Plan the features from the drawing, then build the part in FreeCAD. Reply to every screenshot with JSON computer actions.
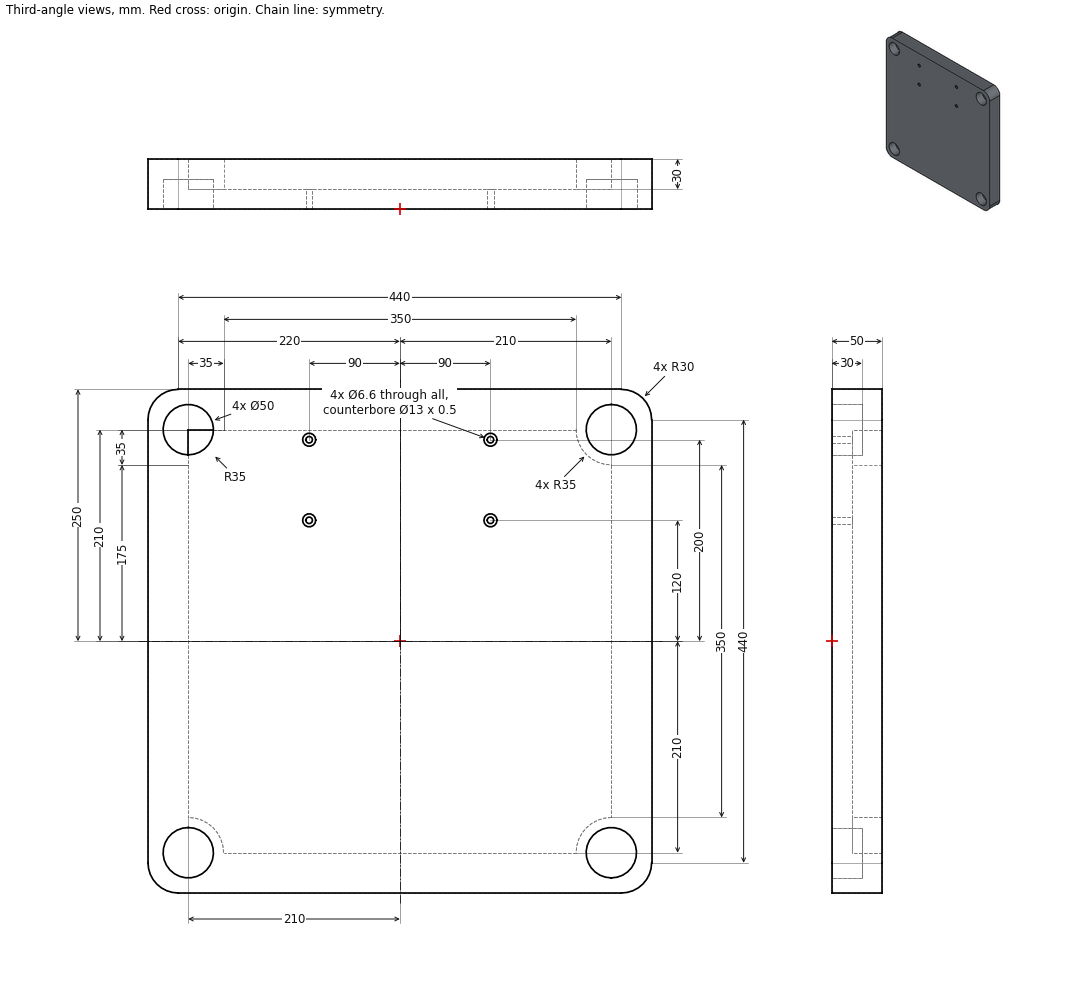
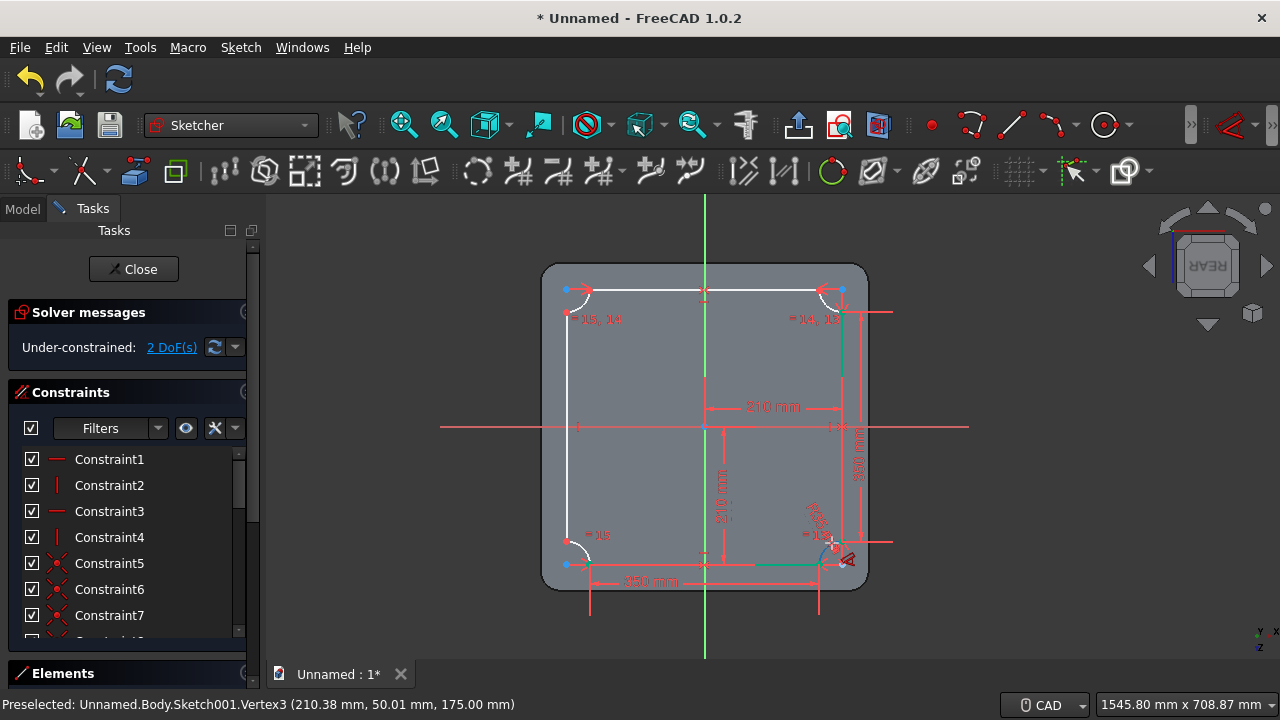
{"action": "left_click", "coordinate": [819, 290]}
{"action": "left_click", "coordinate": [671, 359]}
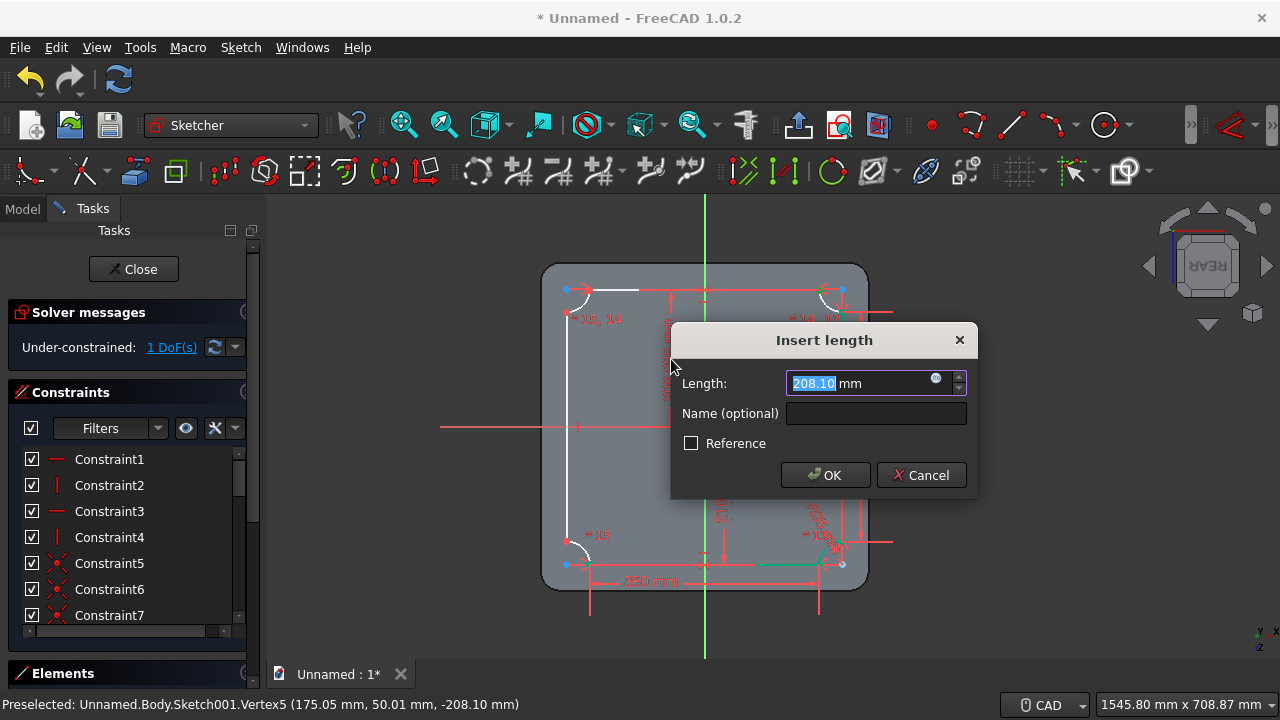
{"action": "type", "text": "210"}
{"action": "key", "text": "Return"}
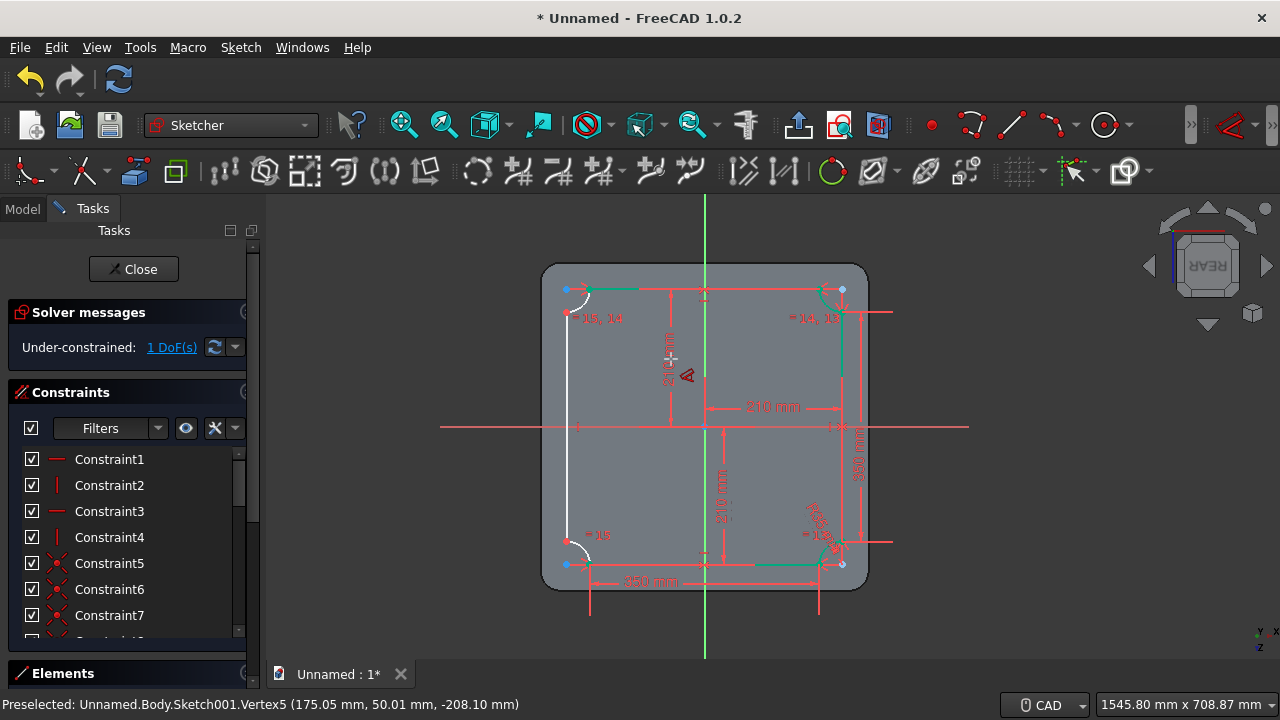
{"action": "left_click", "coordinate": [567, 312]}
{"action": "left_click", "coordinate": [636, 461]}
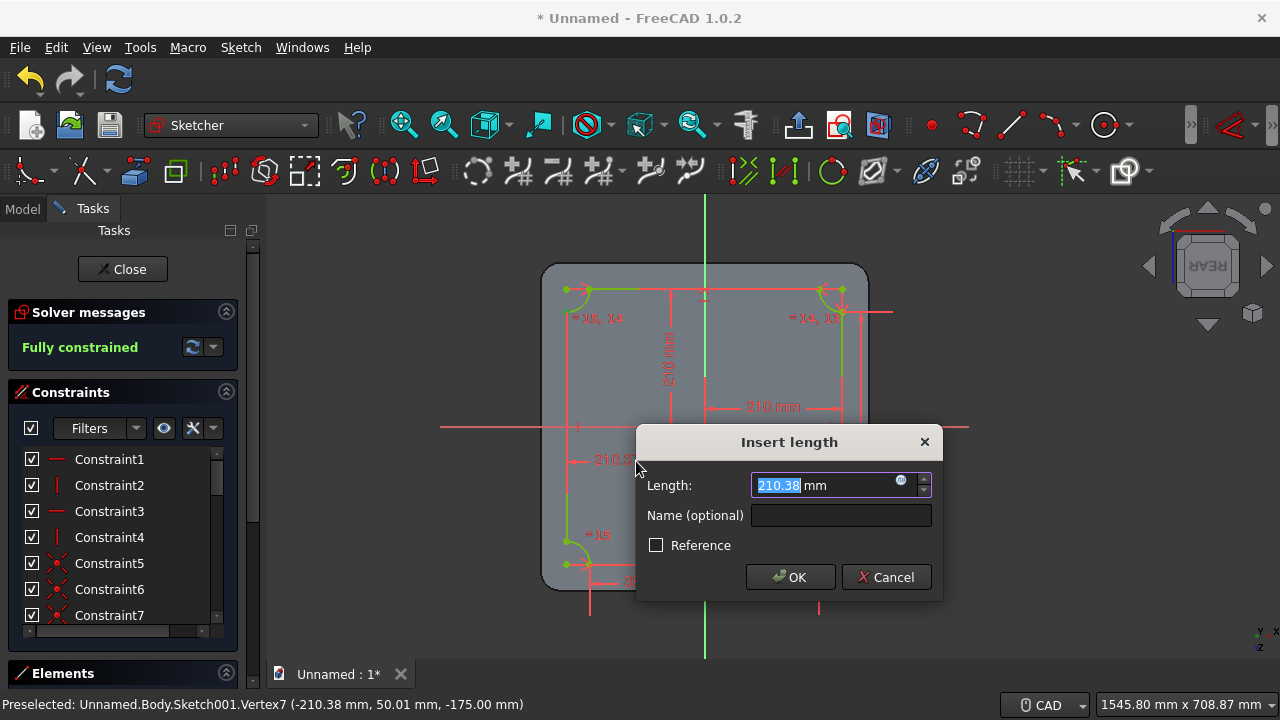
{"action": "type", "text": "210"}
{"action": "key", "text": "Return"}
{"action": "key", "text": "Escape"}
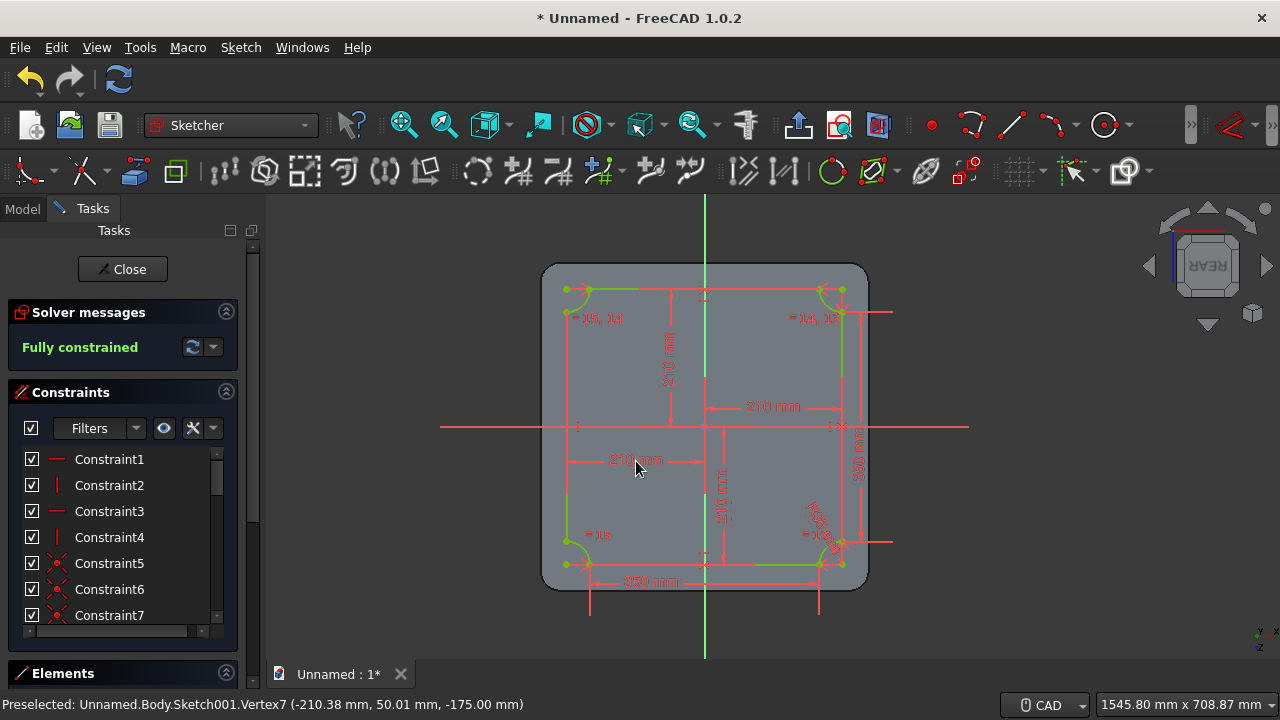
{"action": "left_click", "coordinate": [123, 269]}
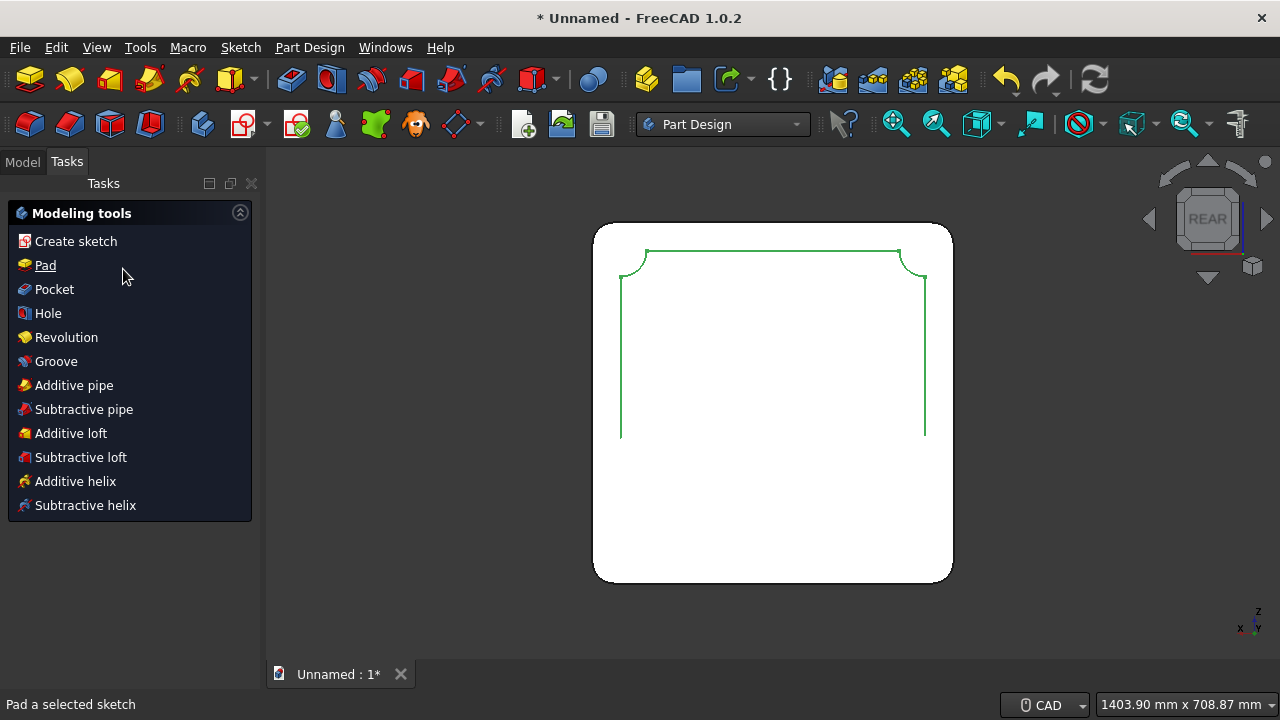
{"action": "left_click", "coordinate": [292, 80]}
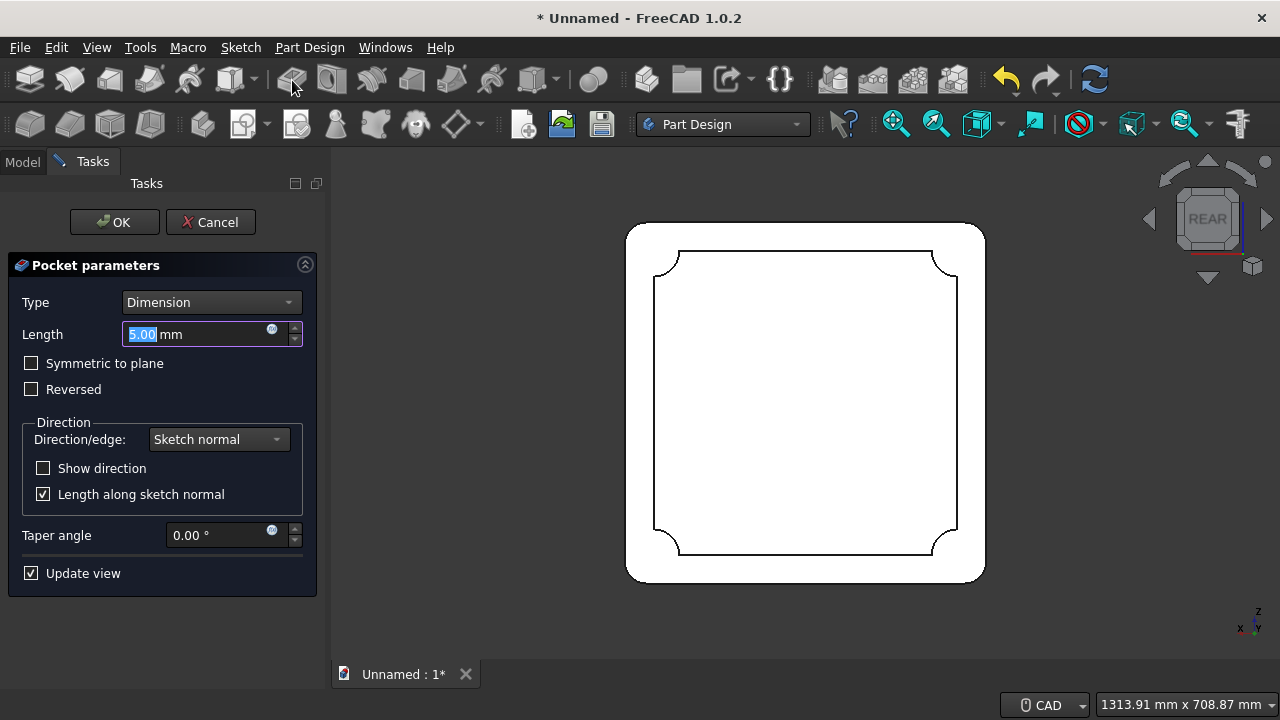
{"action": "type", "text": "30"}
{"action": "key", "text": "Tab"}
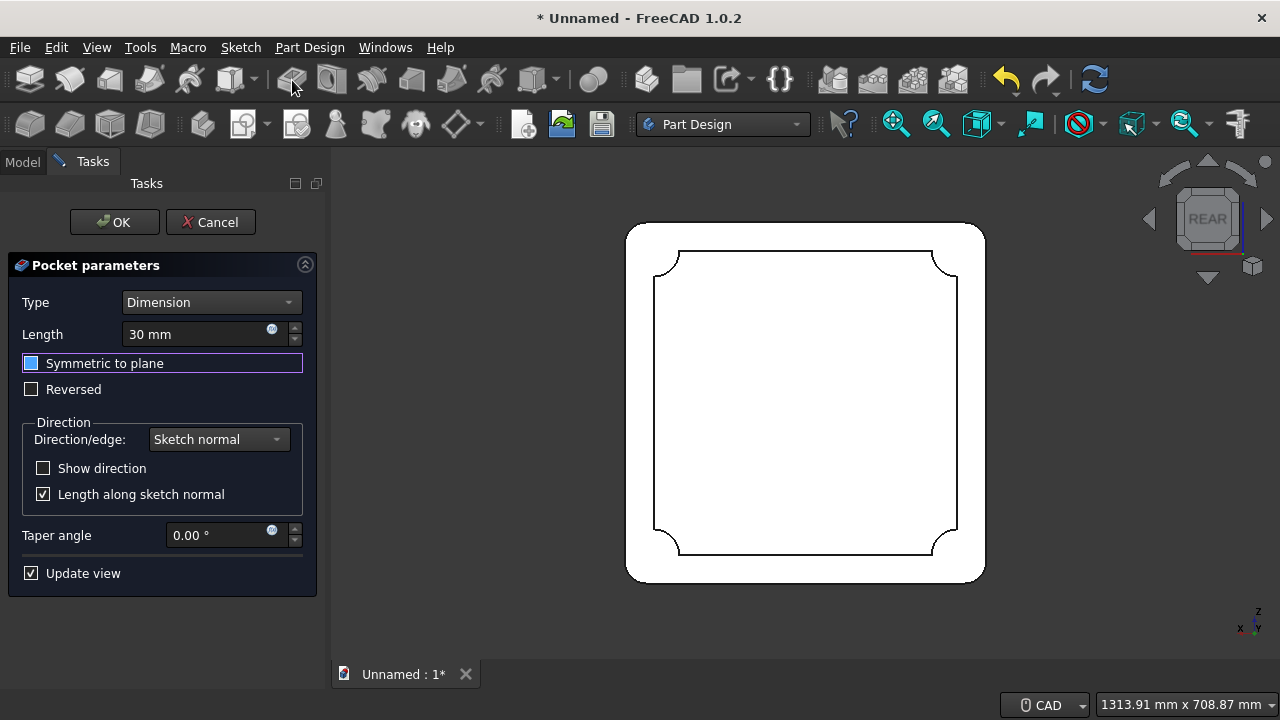
{"action": "left_click", "coordinate": [115, 222]}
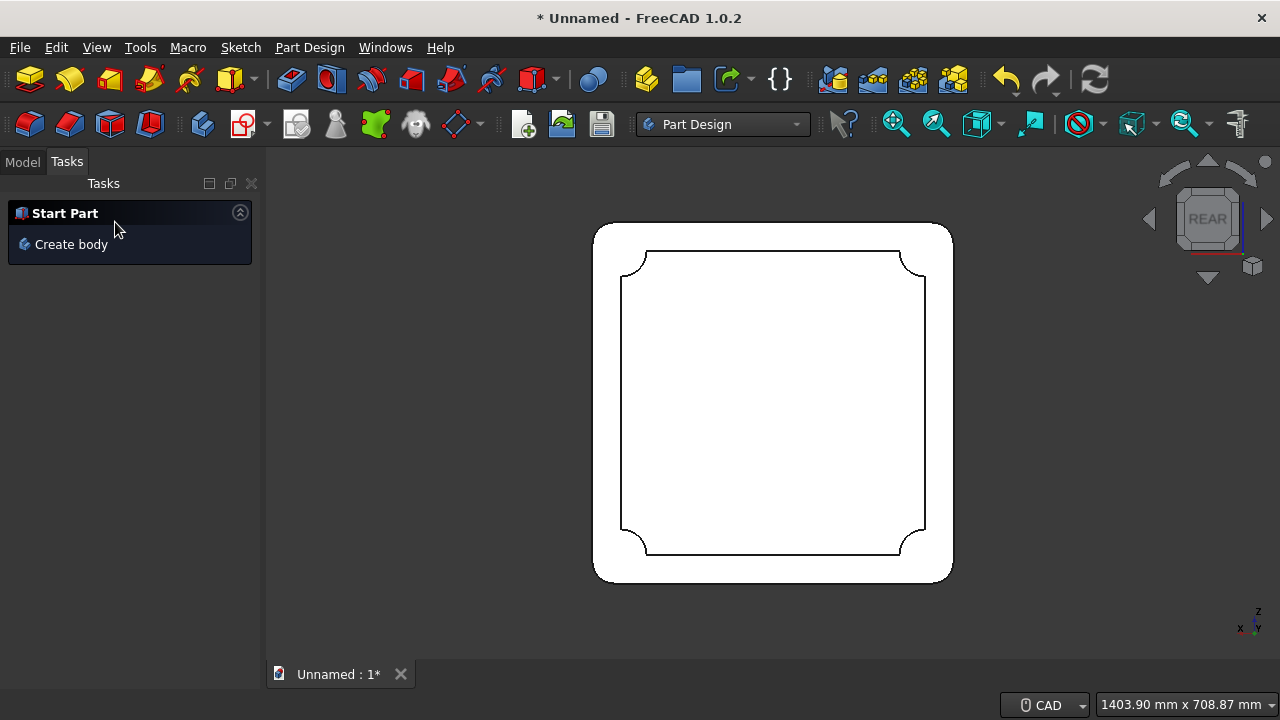
{"action": "key", "text": "0"}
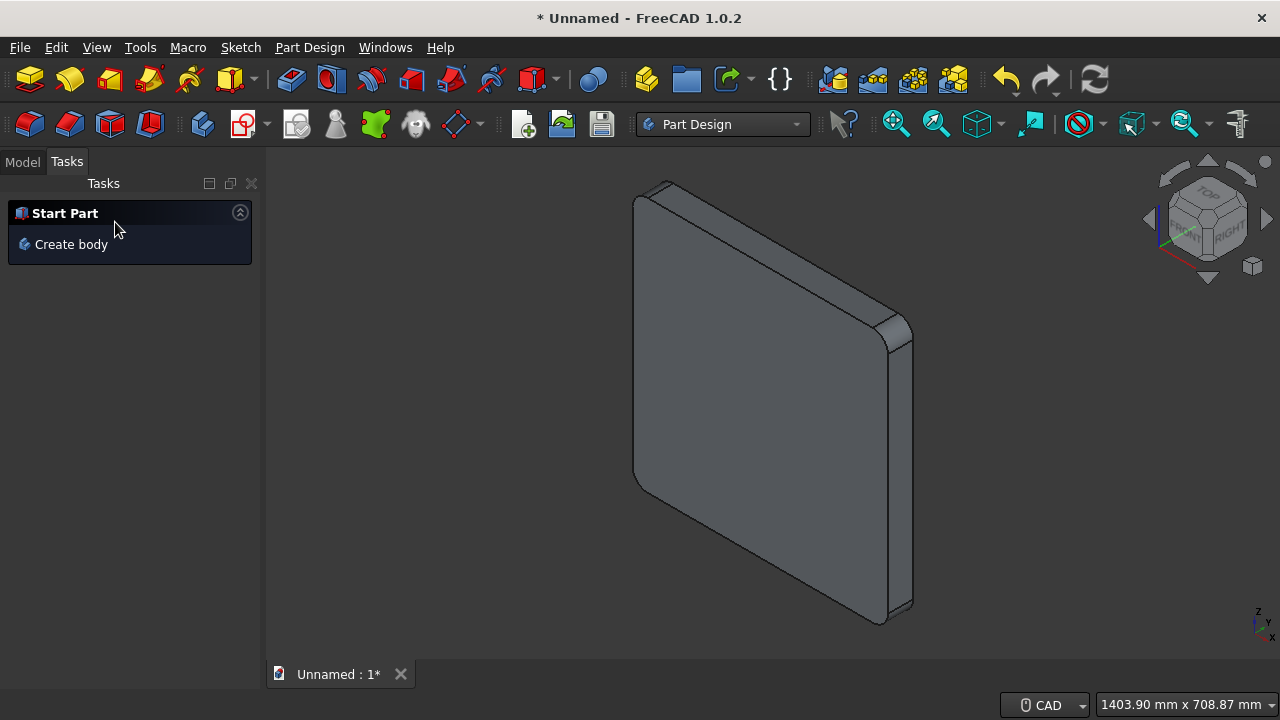
{"action": "left_click", "coordinate": [760, 409]}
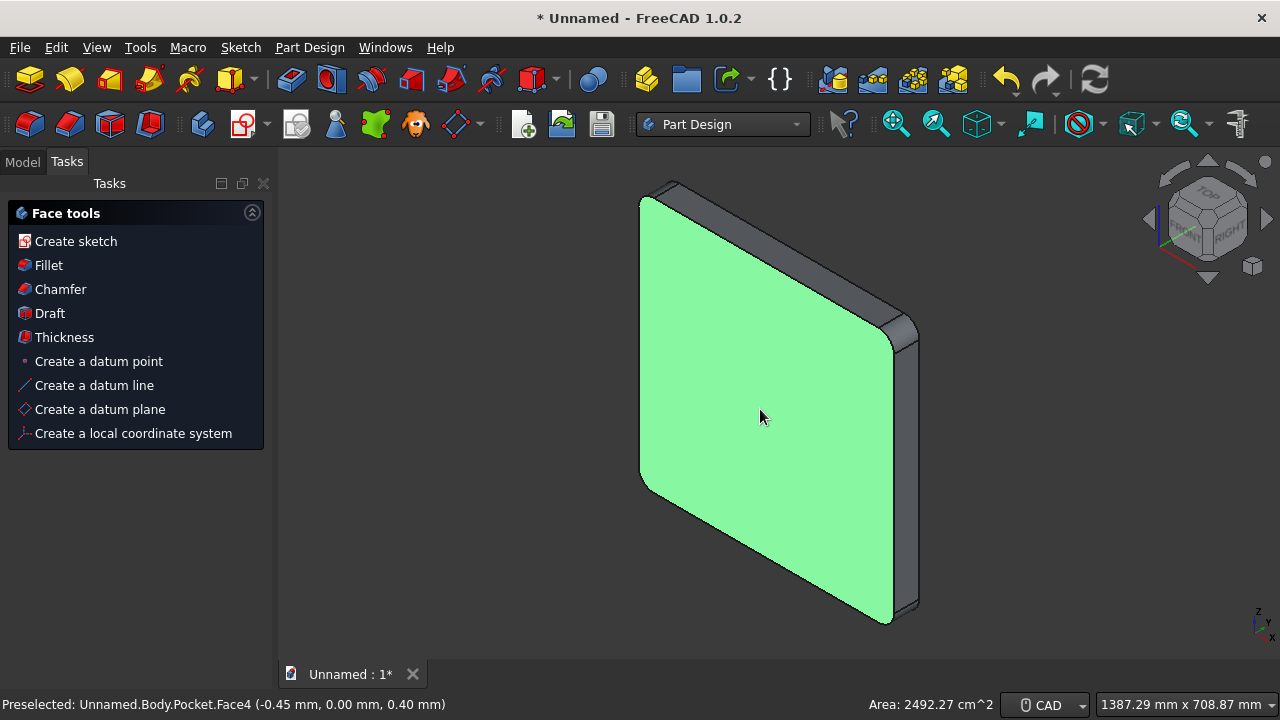
{"action": "left_click", "coordinate": [244, 124]}